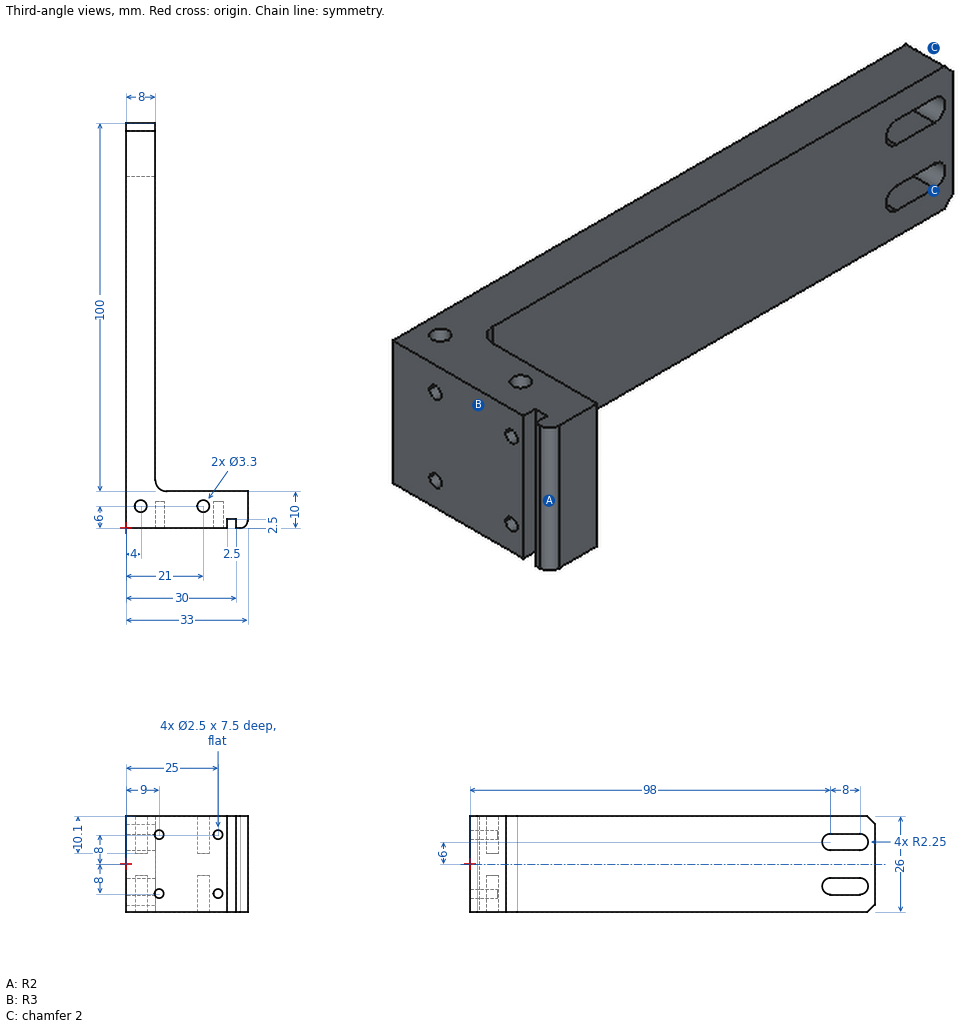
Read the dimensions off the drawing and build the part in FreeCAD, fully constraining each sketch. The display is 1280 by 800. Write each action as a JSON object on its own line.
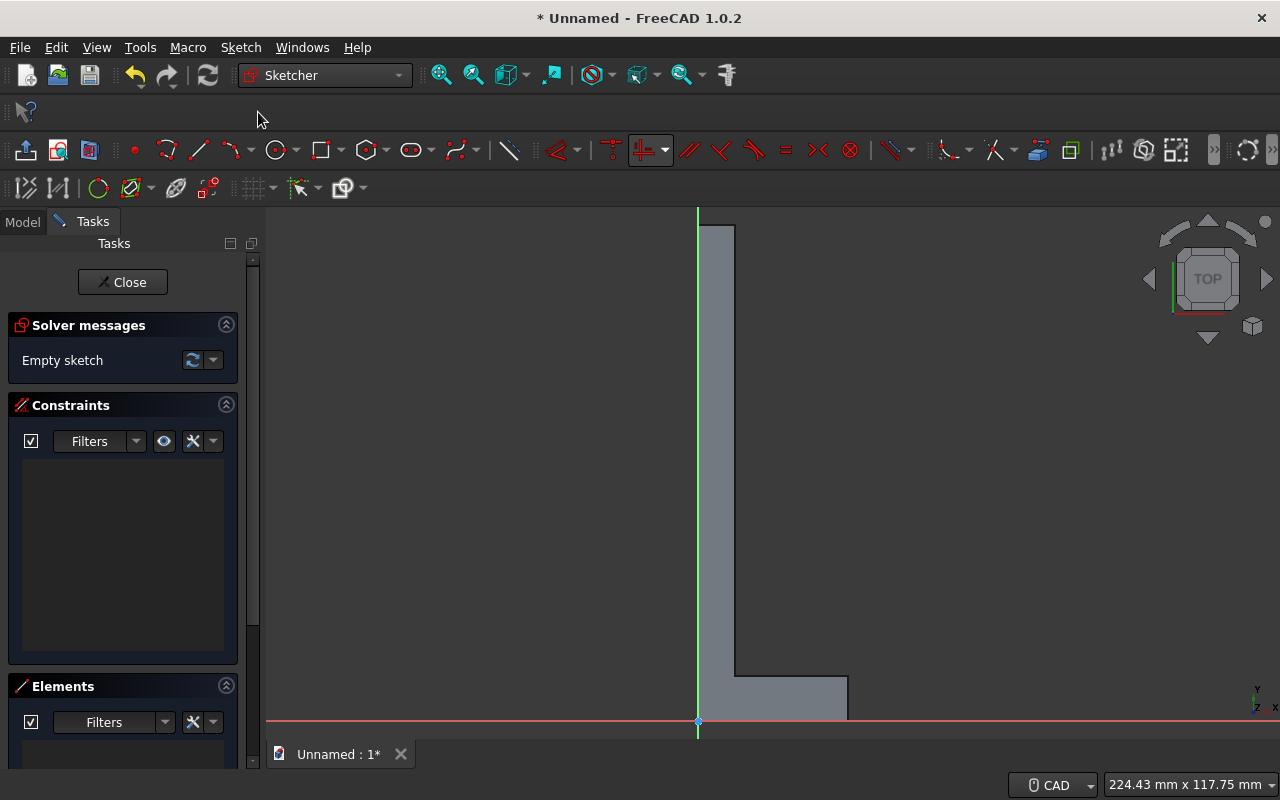
{"action": "scroll", "coordinate": [704, 473], "scroll_direction": "down", "scroll_amount": 5}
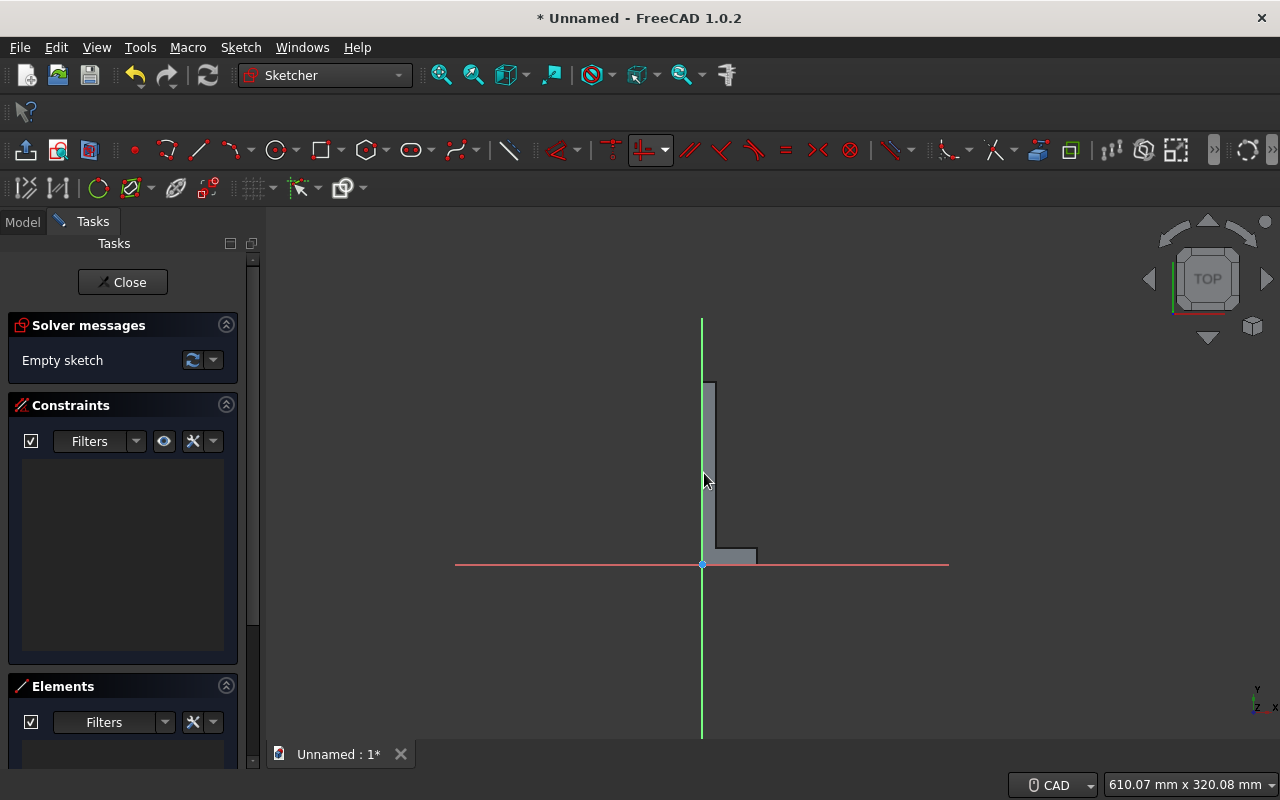
{"action": "scroll", "coordinate": [752, 567], "scroll_direction": "up", "scroll_amount": 15}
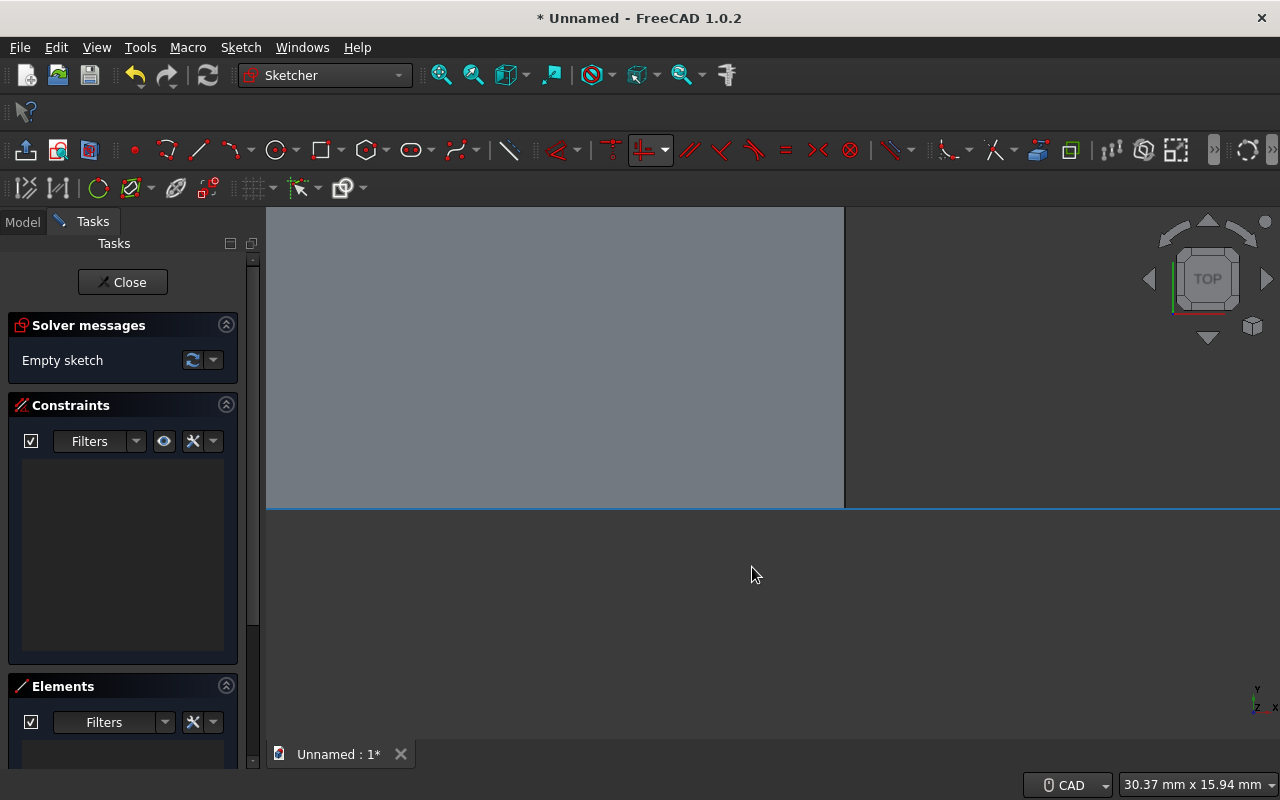
{"action": "scroll", "coordinate": [703, 465], "scroll_direction": "up", "scroll_amount": 7}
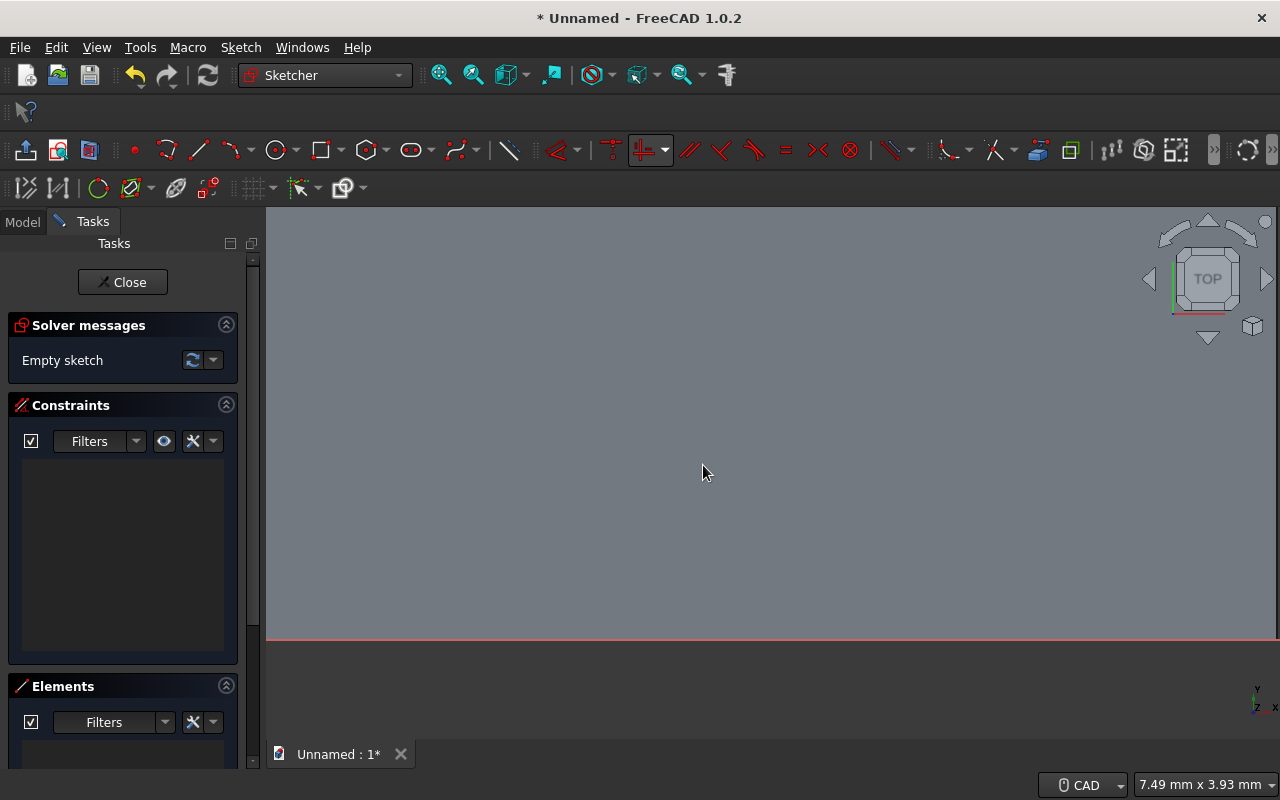
{"action": "left_click", "coordinate": [322, 150]}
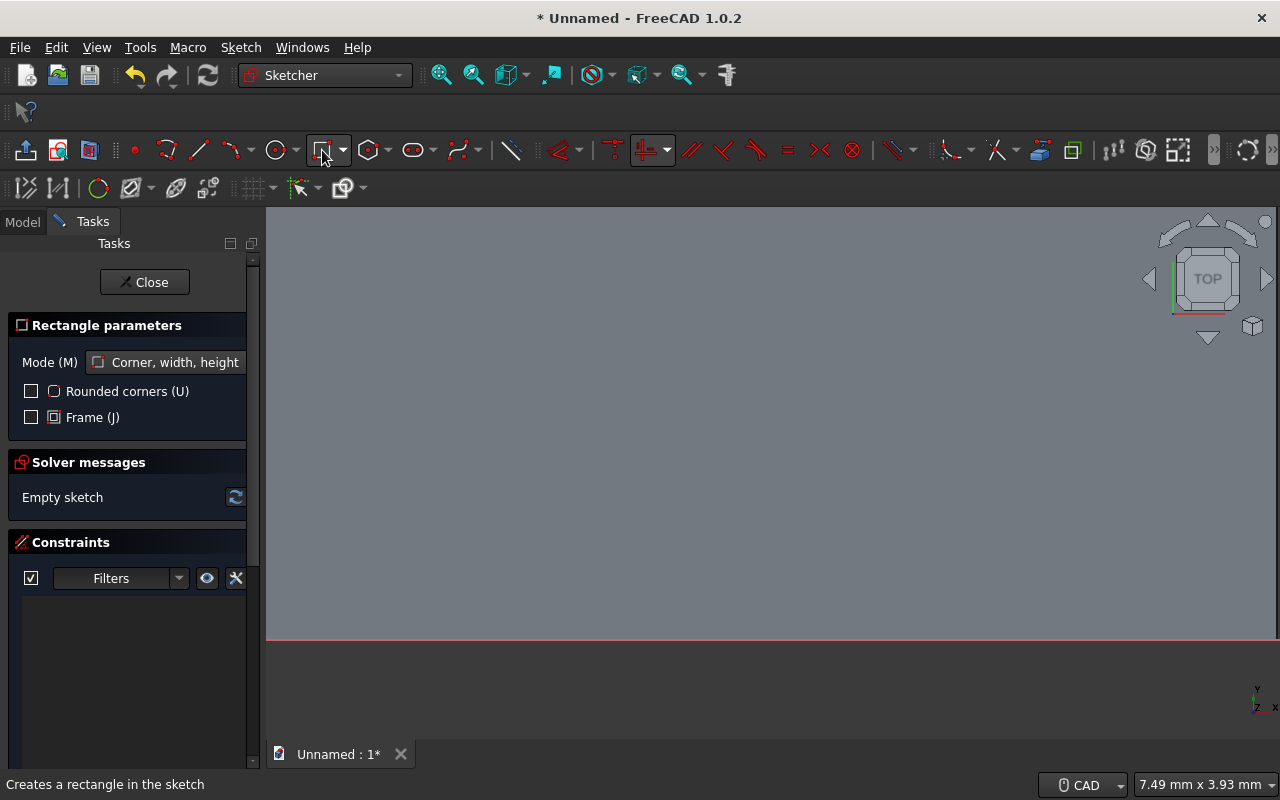
{"action": "left_click", "coordinate": [533, 302]}
{"action": "left_click", "coordinate": [871, 640]}
{"action": "key", "text": "Escape"}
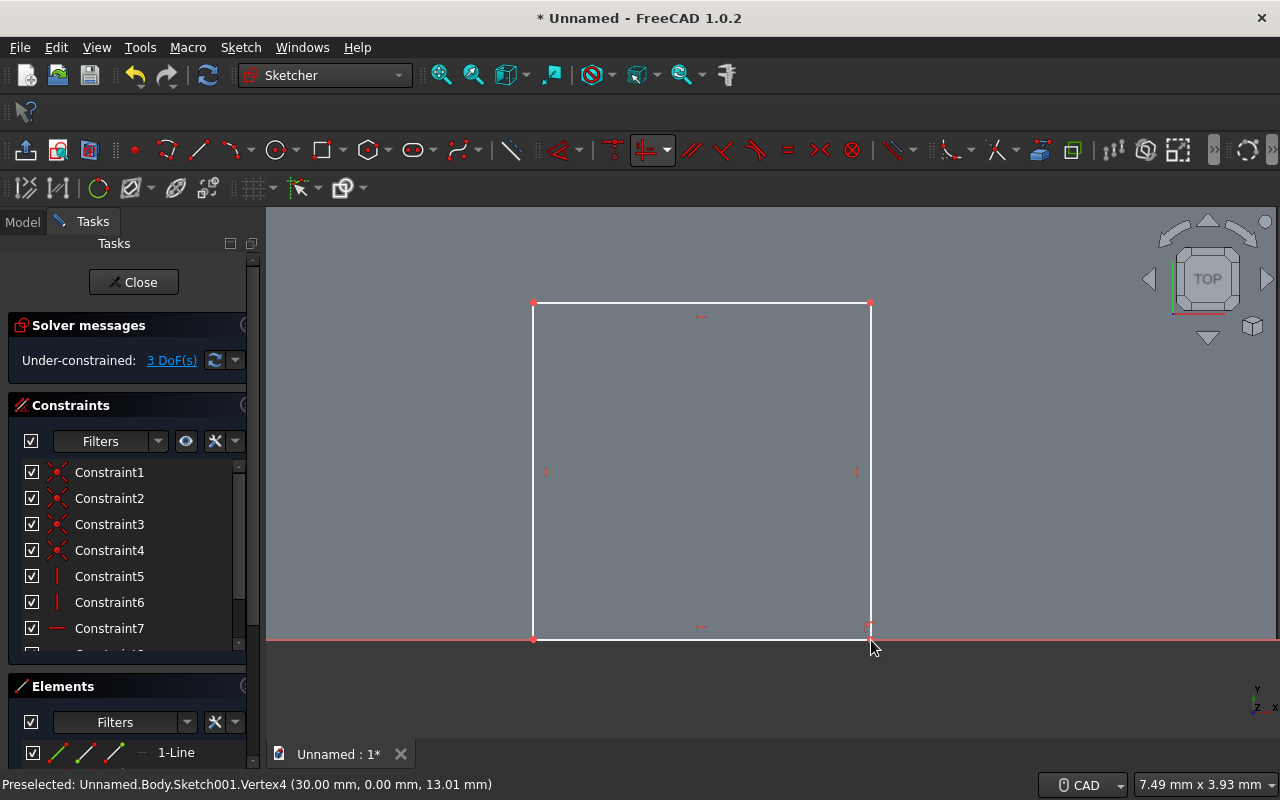
{"action": "left_click", "coordinate": [558, 150]}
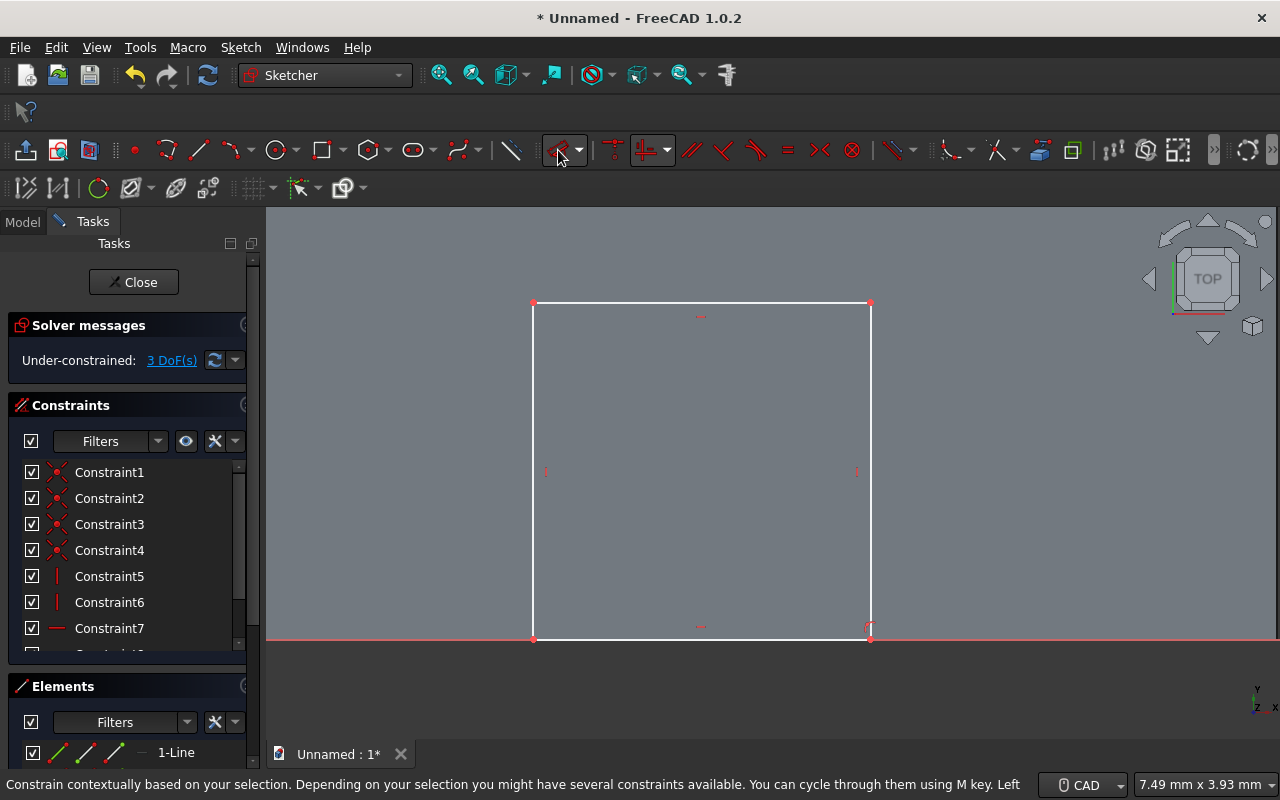
{"action": "left_click", "coordinate": [533, 404]}
{"action": "left_click", "coordinate": [499, 471]}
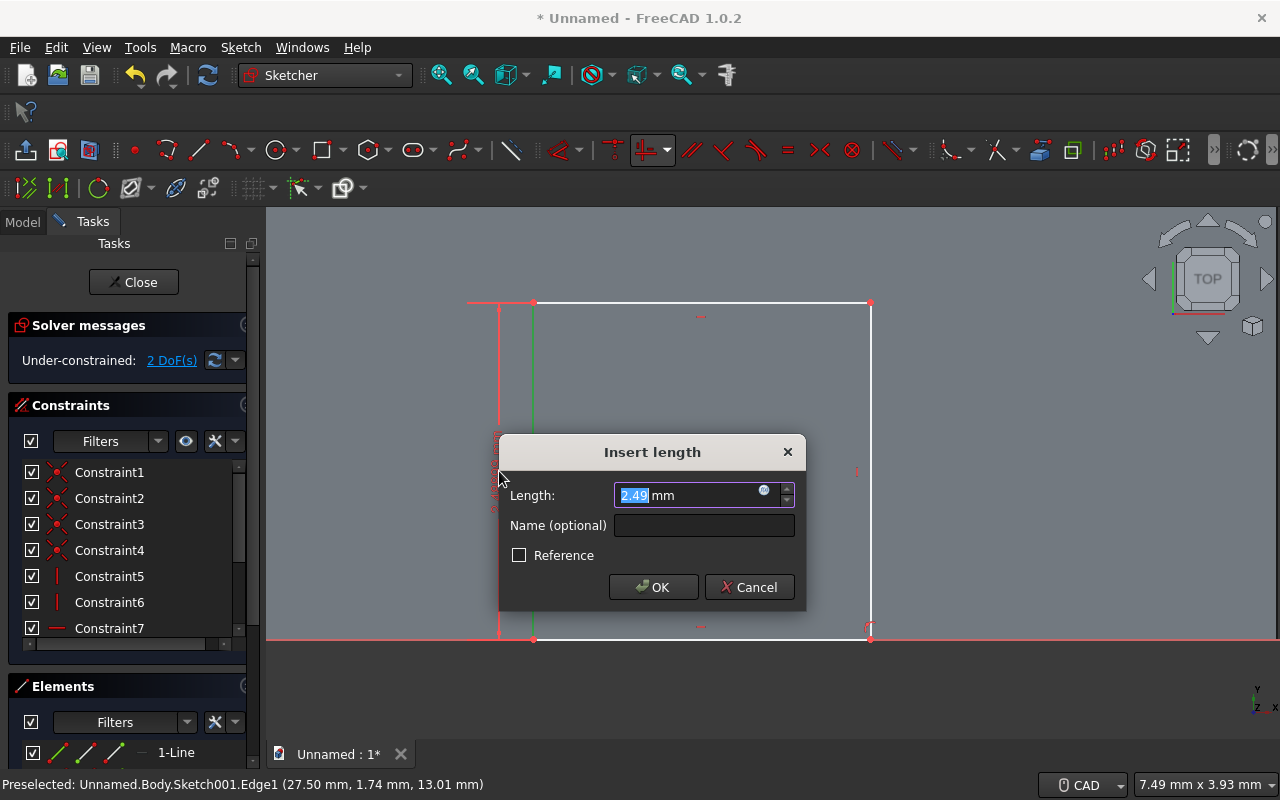
{"action": "type", "text": "2.5"}
{"action": "key", "text": "Return"}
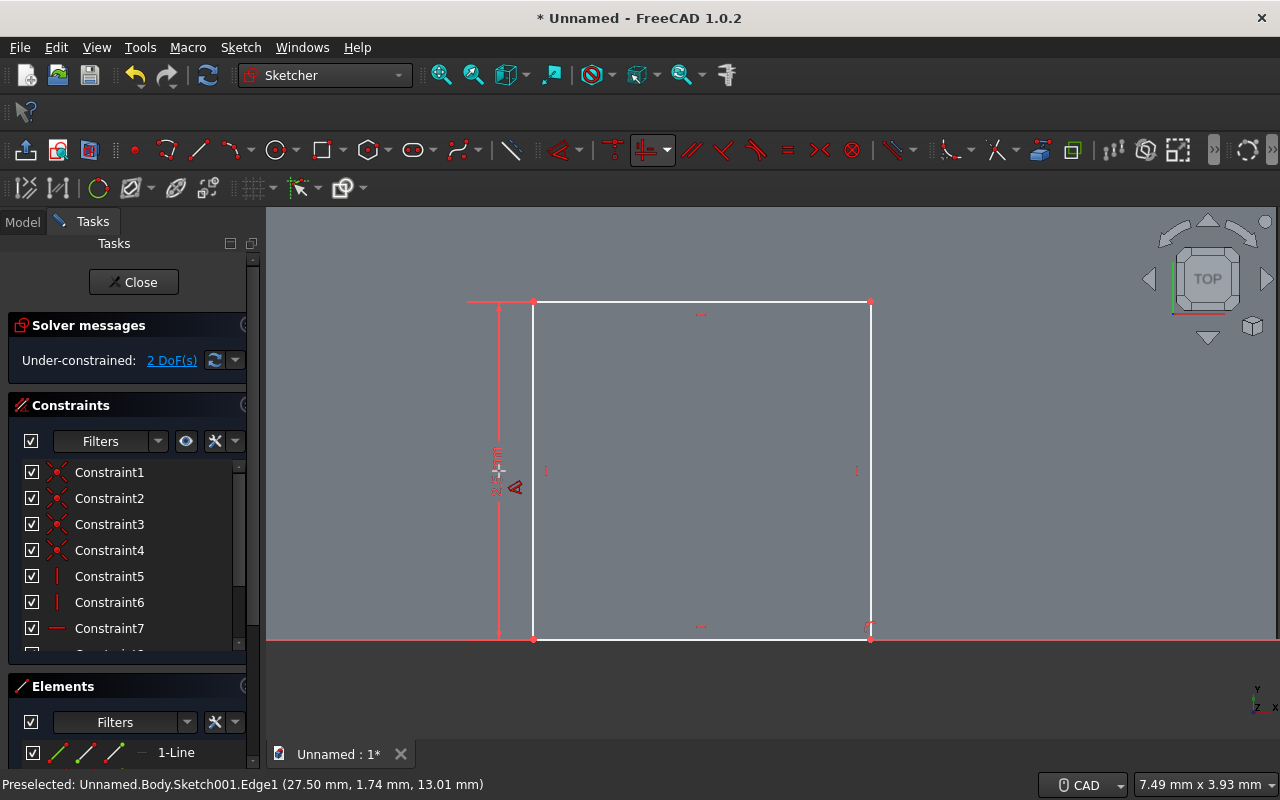
{"action": "left_click", "coordinate": [634, 640]}
{"action": "left_click", "coordinate": [702, 674]}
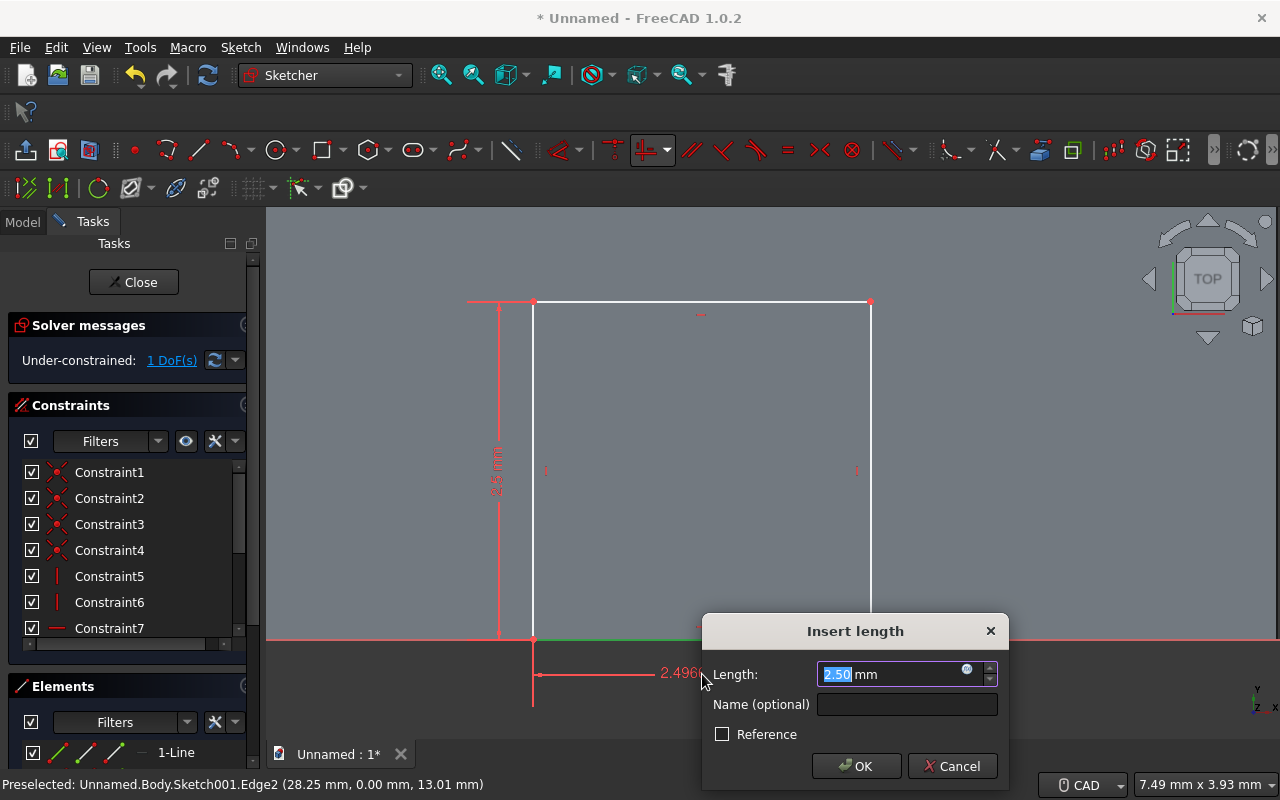
{"action": "type", "text": "2.5"}
{"action": "key", "text": "Return"}